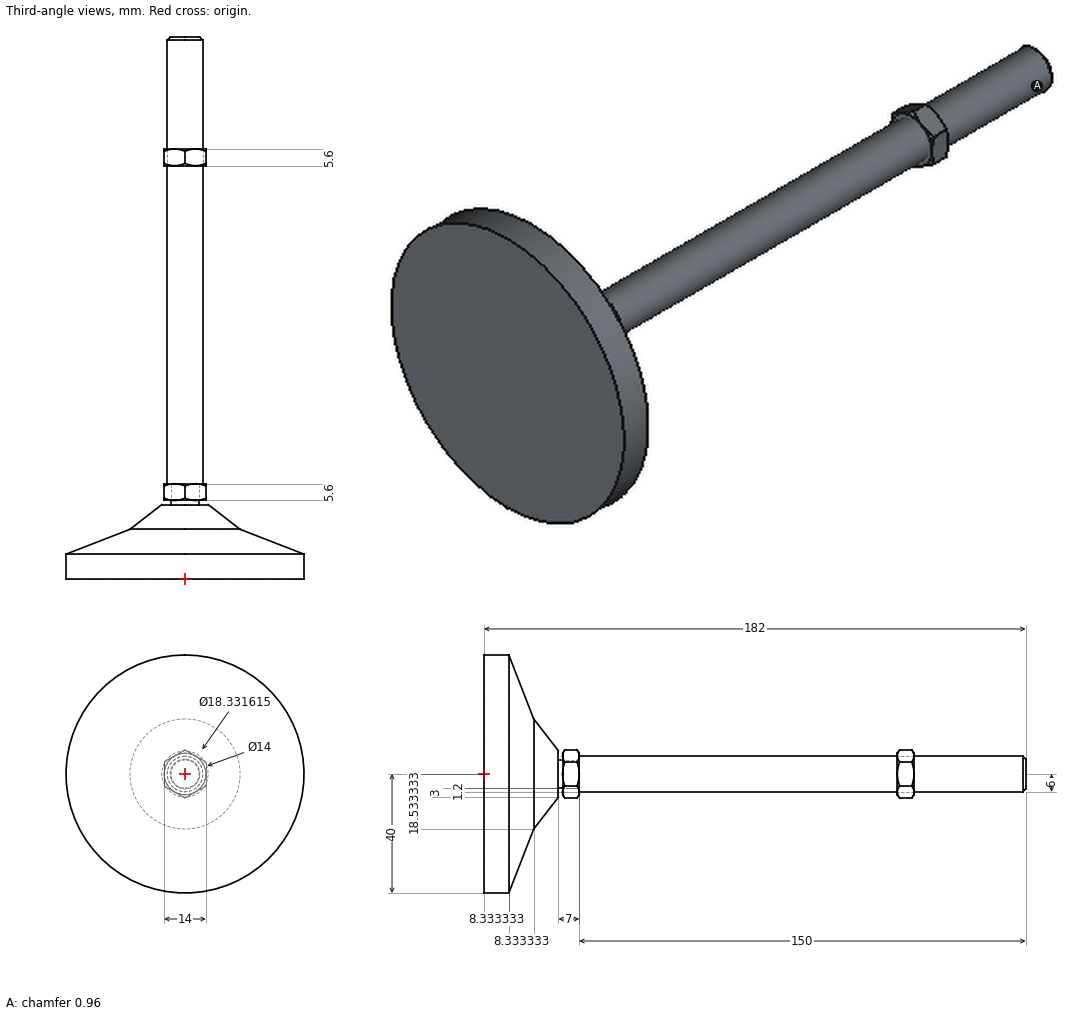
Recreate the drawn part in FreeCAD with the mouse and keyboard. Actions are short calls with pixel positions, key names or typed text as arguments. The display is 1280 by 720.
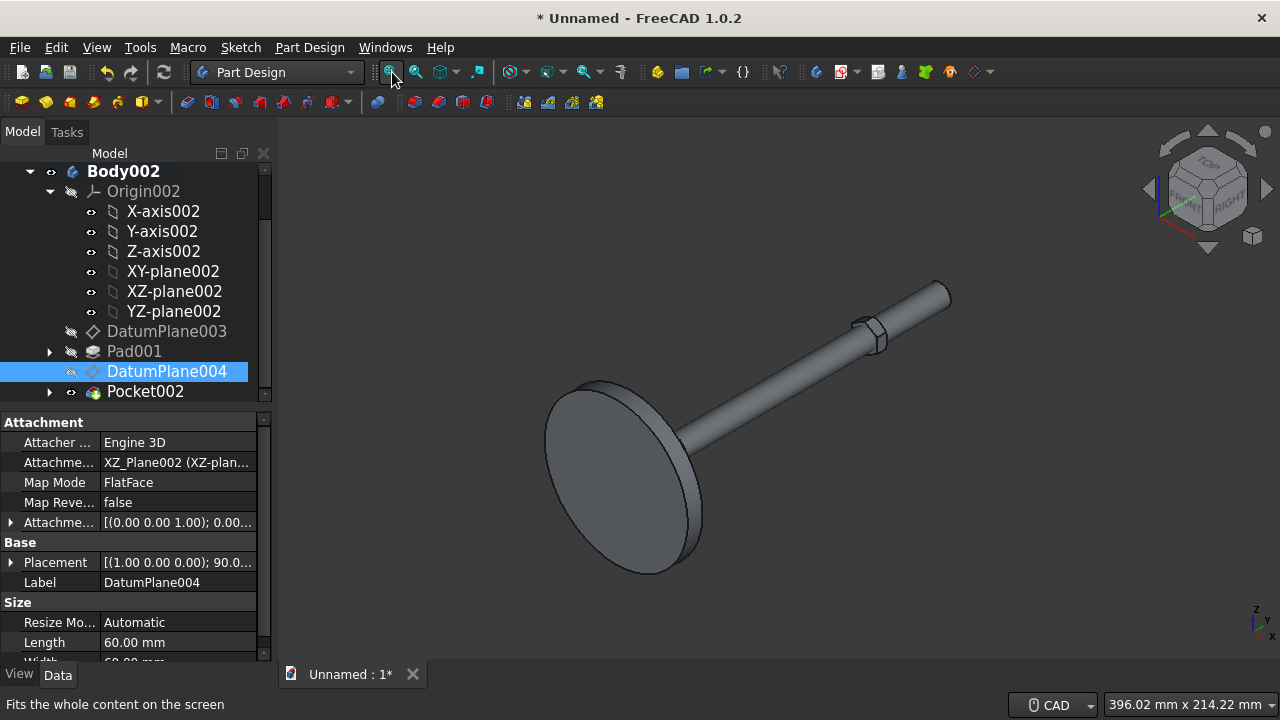
click(392, 72)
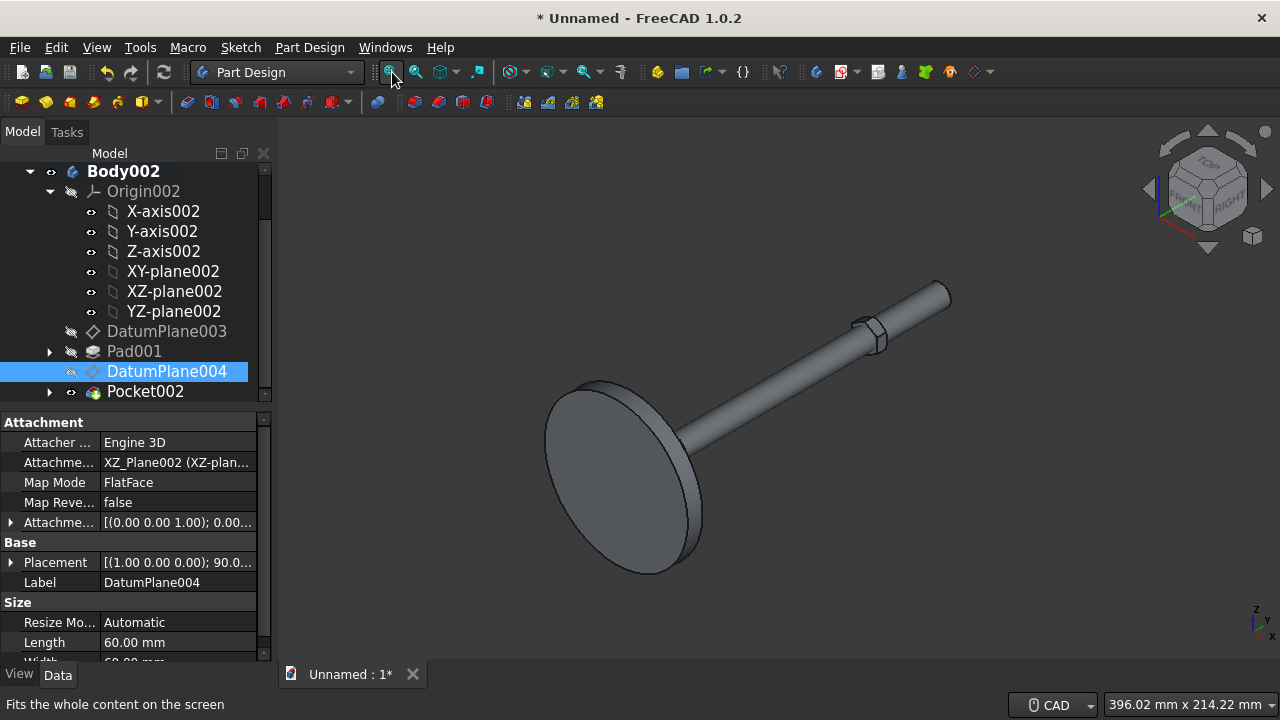
key(1)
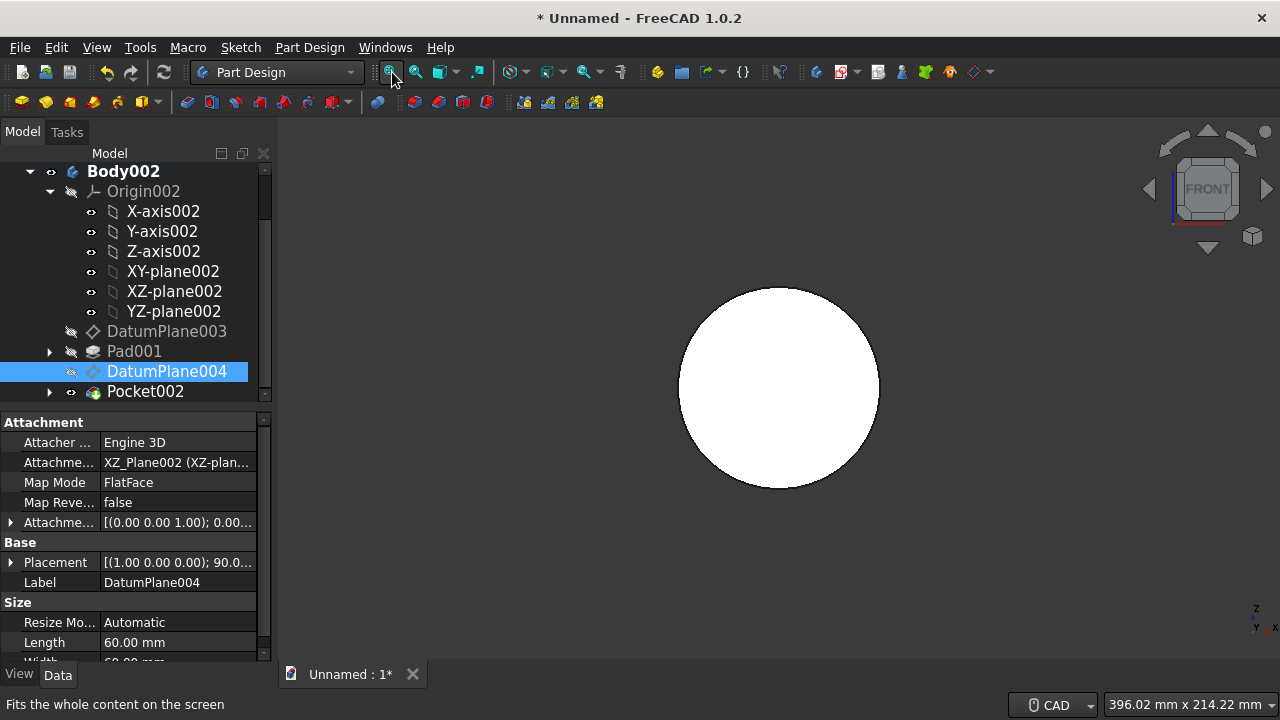
click(392, 72)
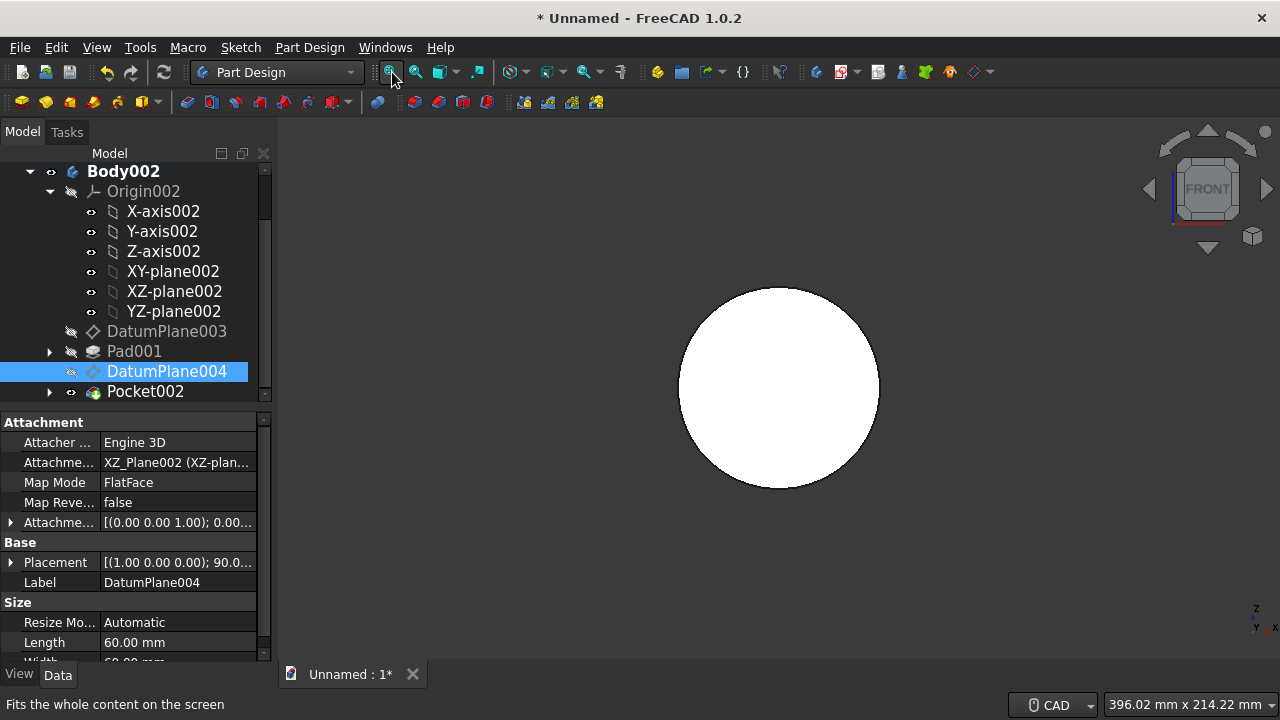
key(2)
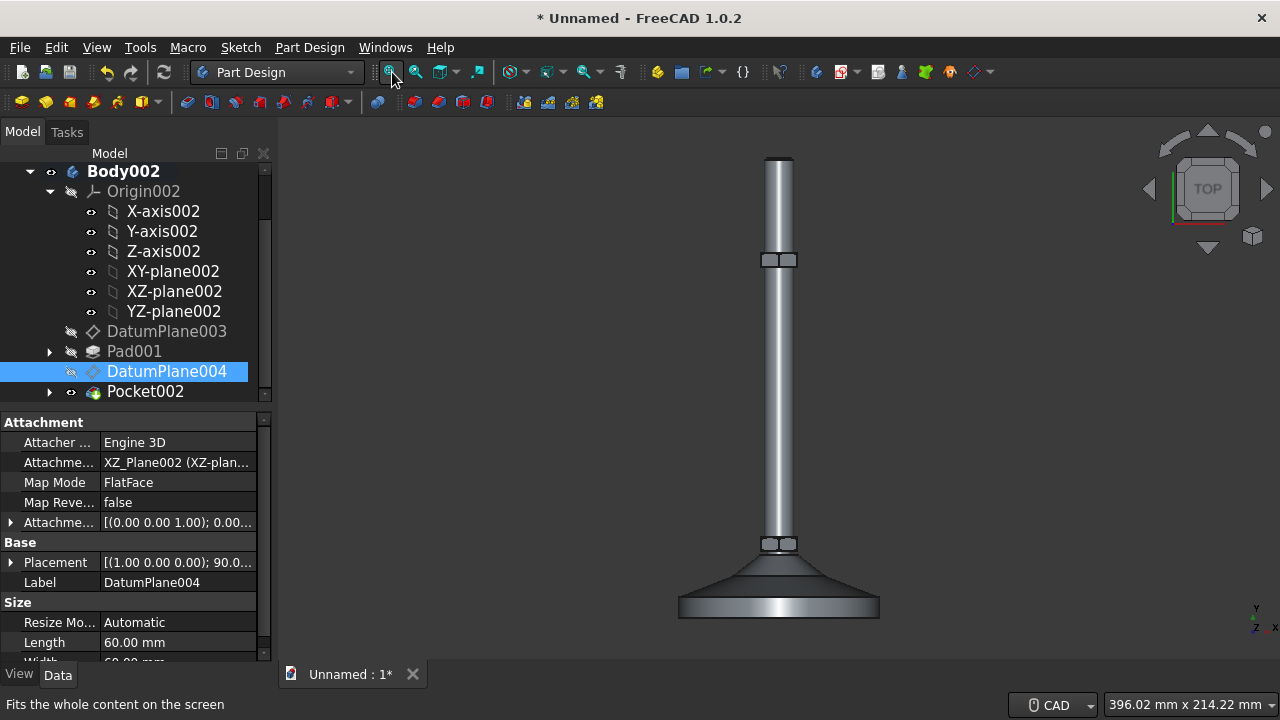
click(392, 72)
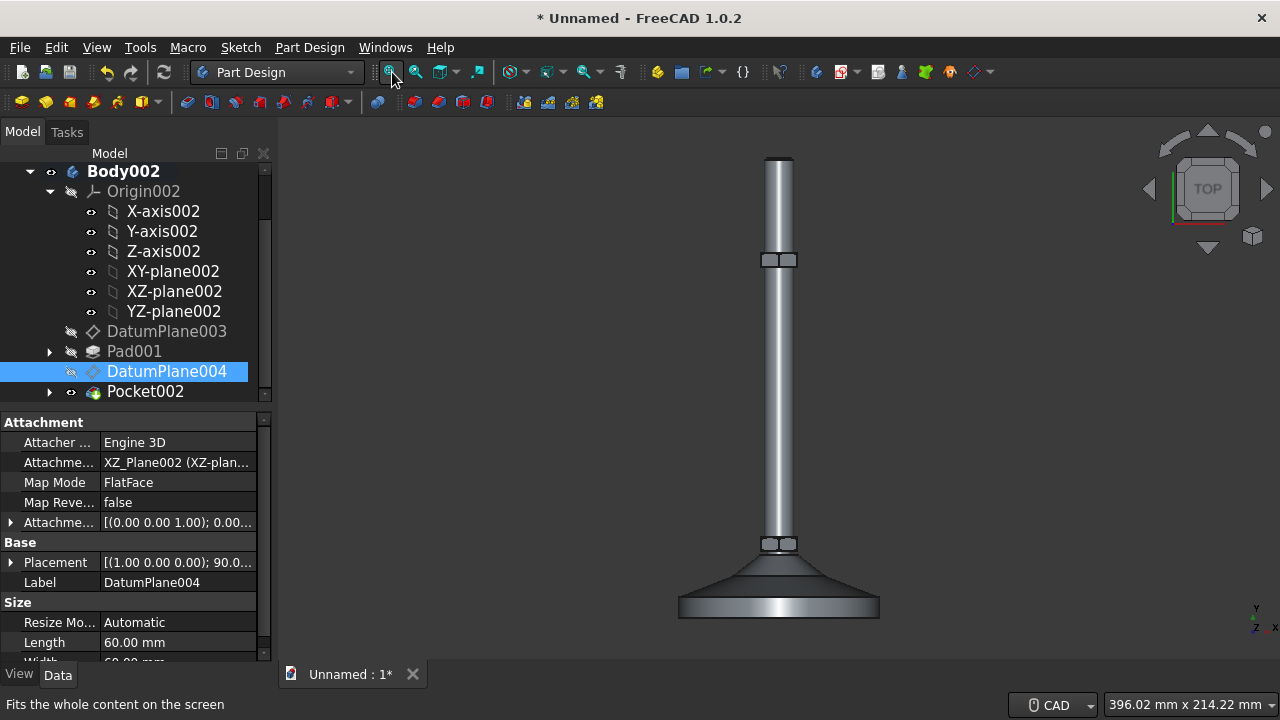
click(136, 292)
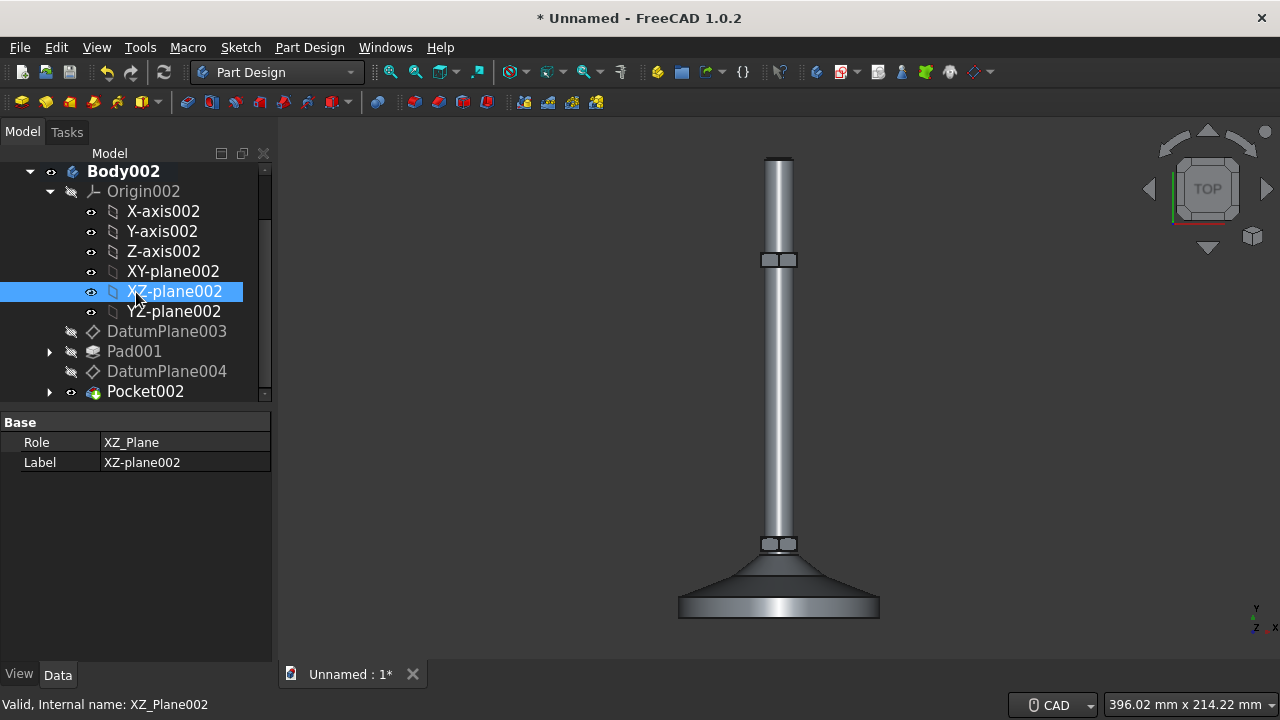
click(974, 72)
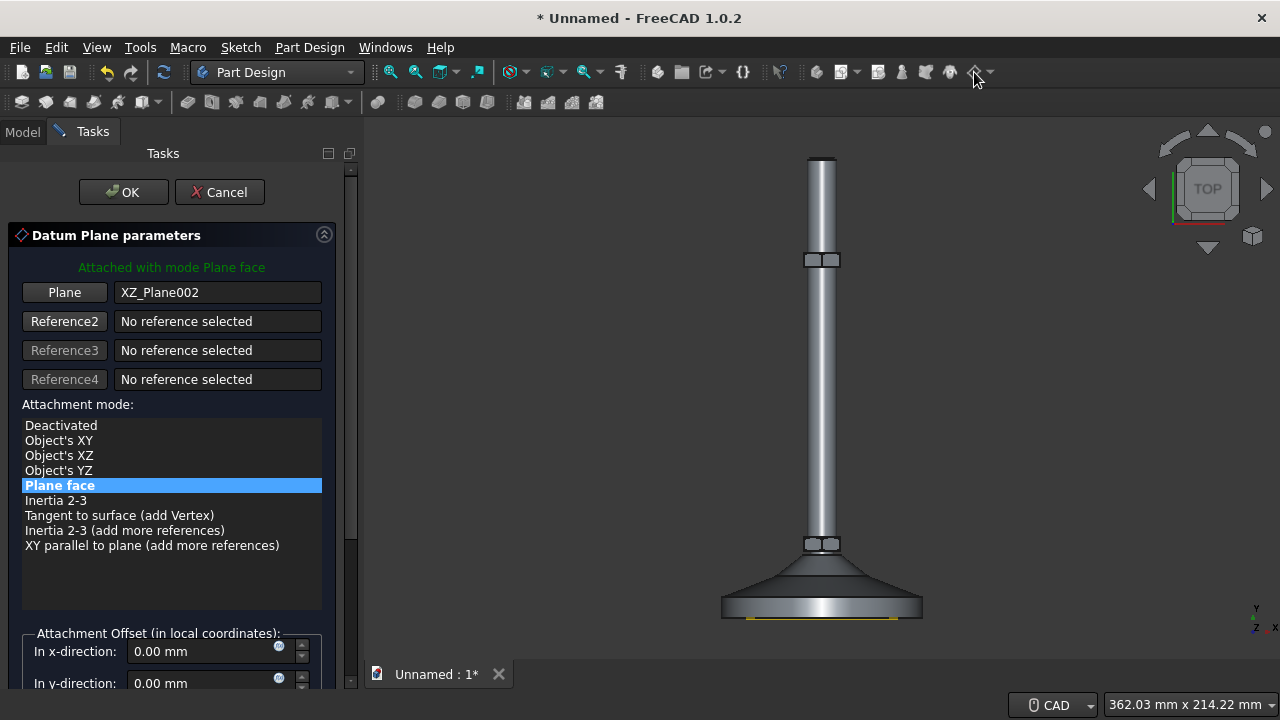
scroll(351, 426, down, 2)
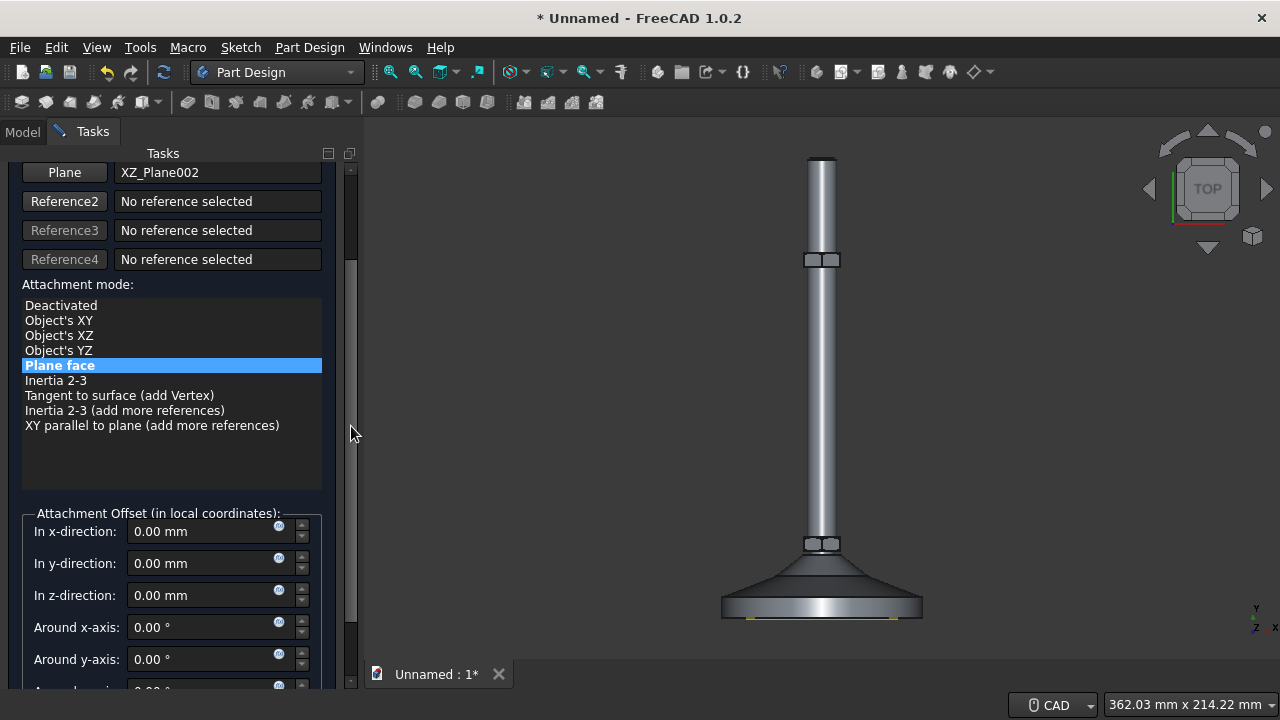
triple_click(210, 595)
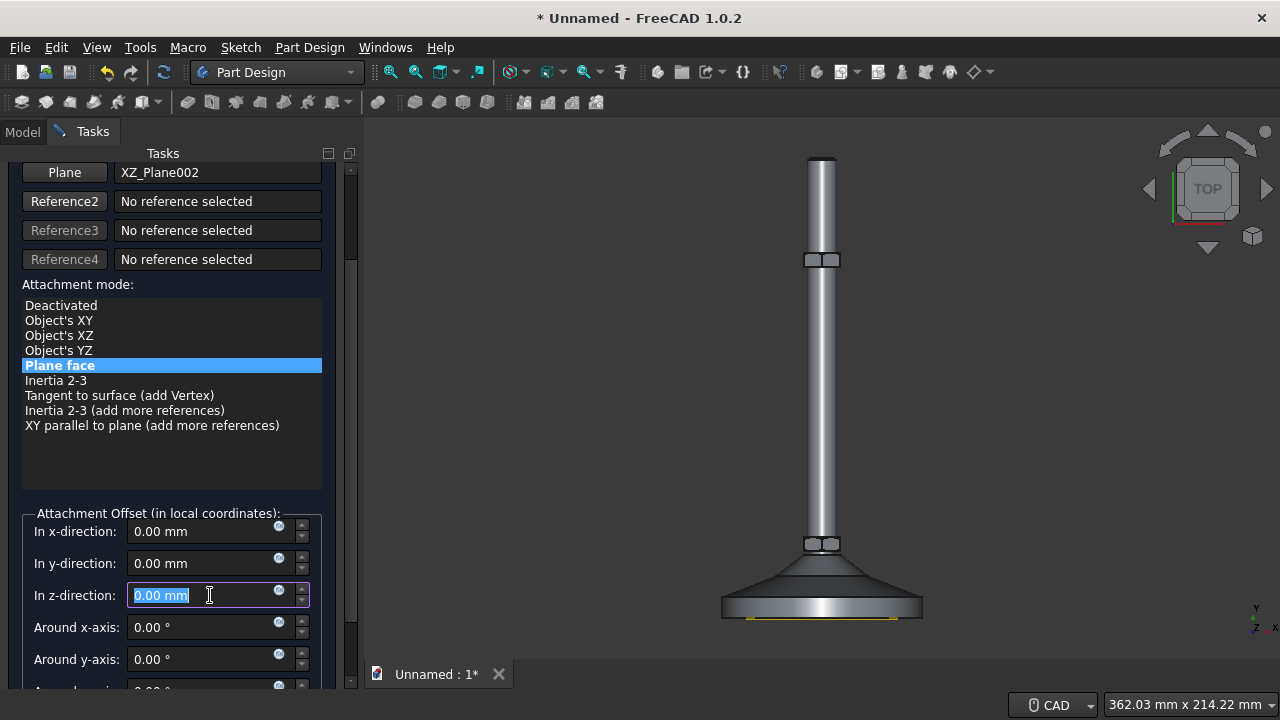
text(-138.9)
key(Tab)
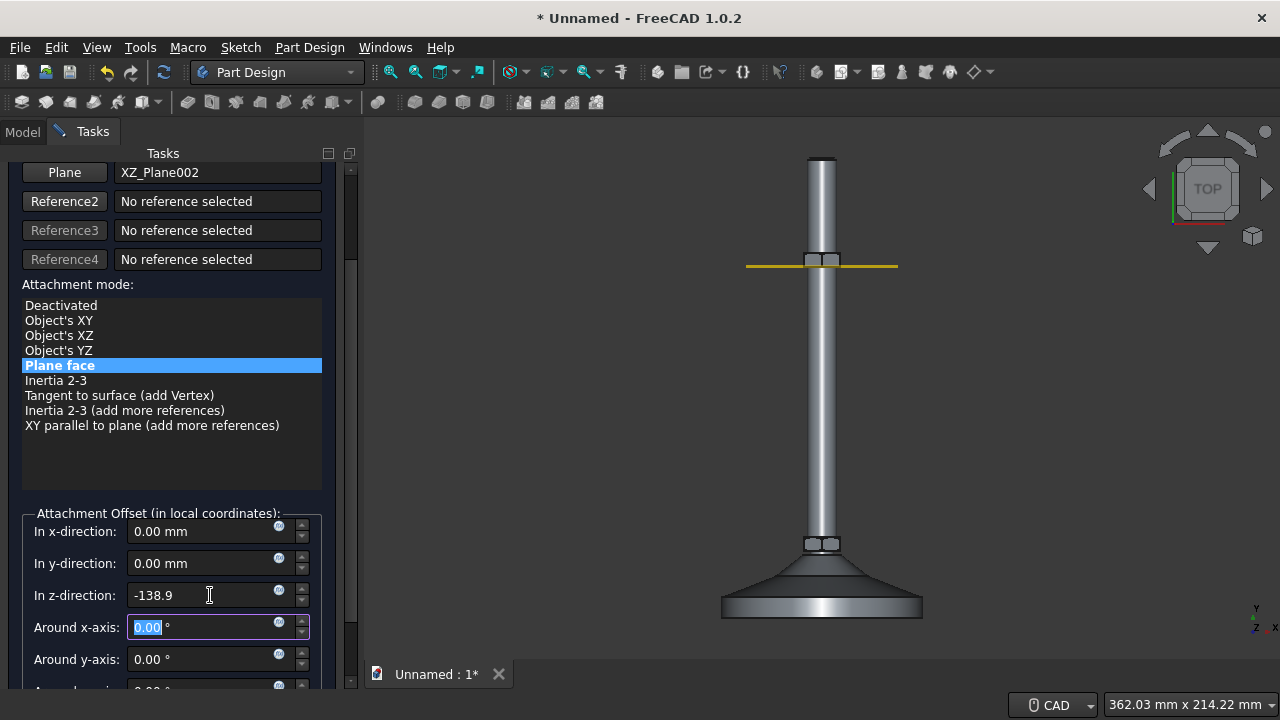
scroll(351, 426, up, 3)